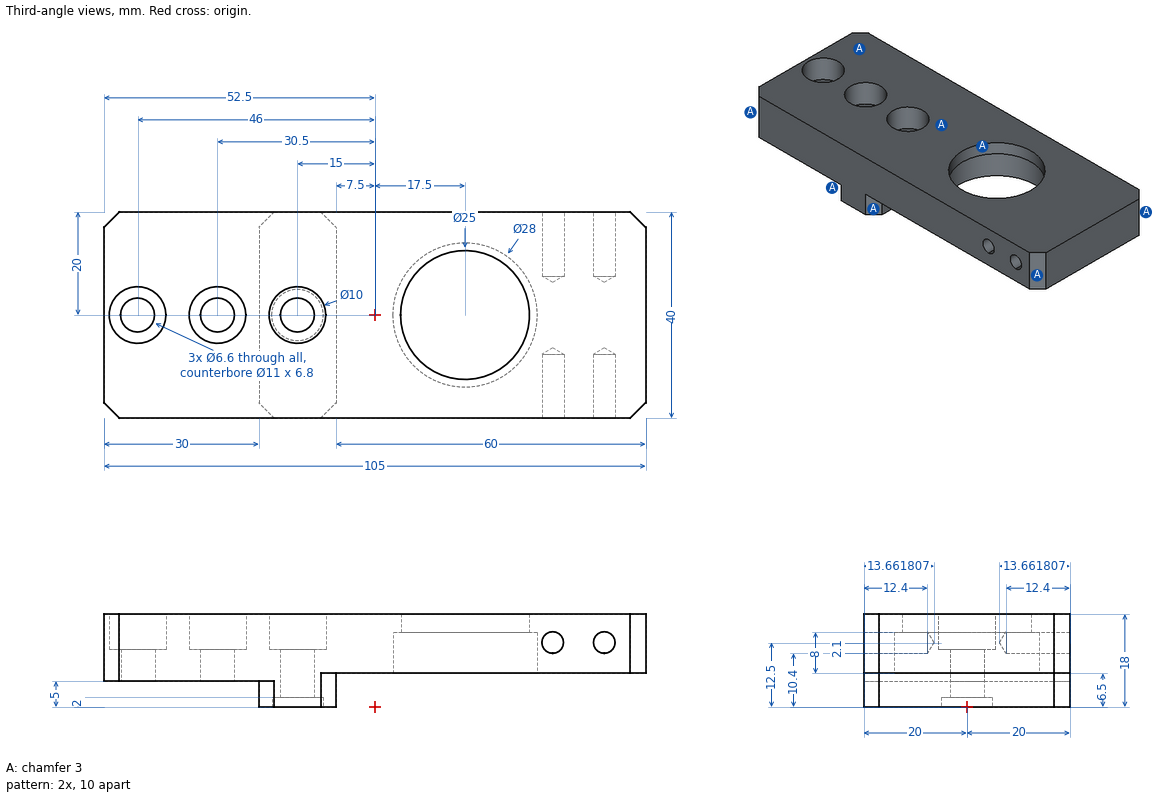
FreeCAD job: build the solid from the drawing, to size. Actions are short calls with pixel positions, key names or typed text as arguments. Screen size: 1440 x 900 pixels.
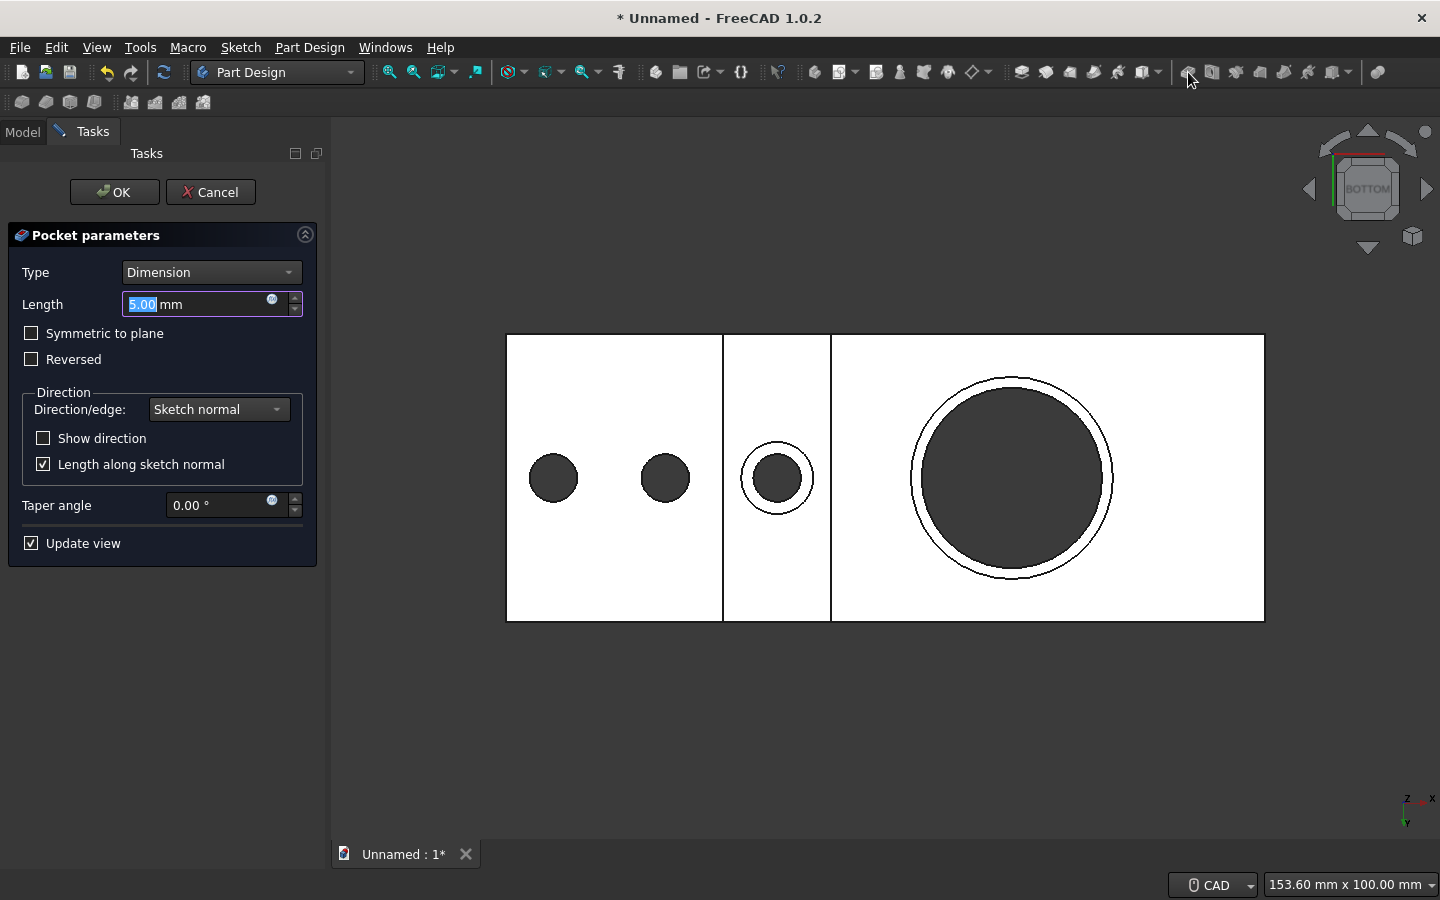
click(212, 272)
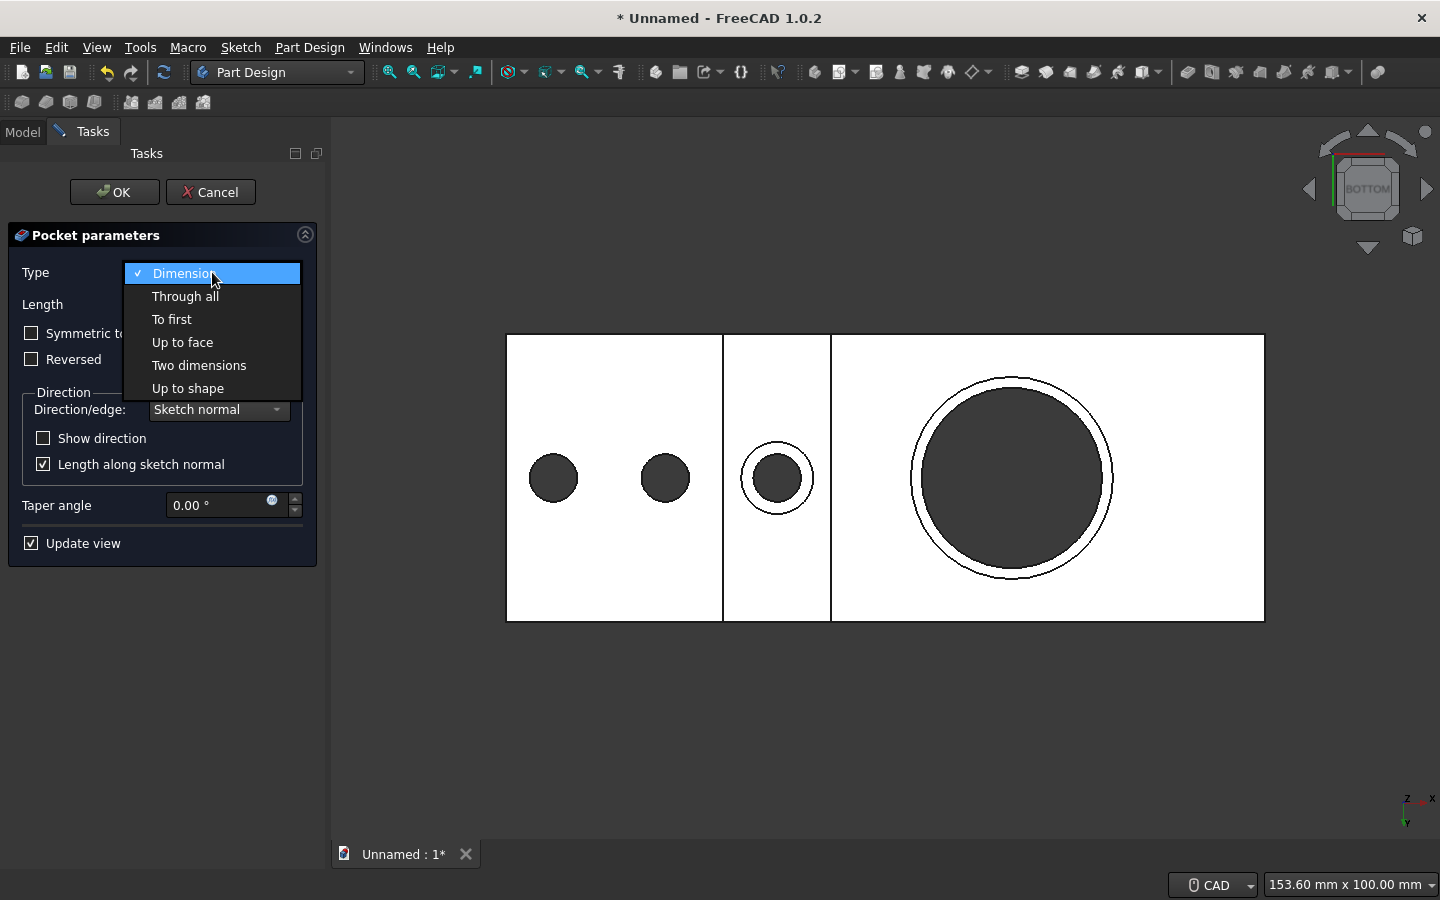
click(212, 296)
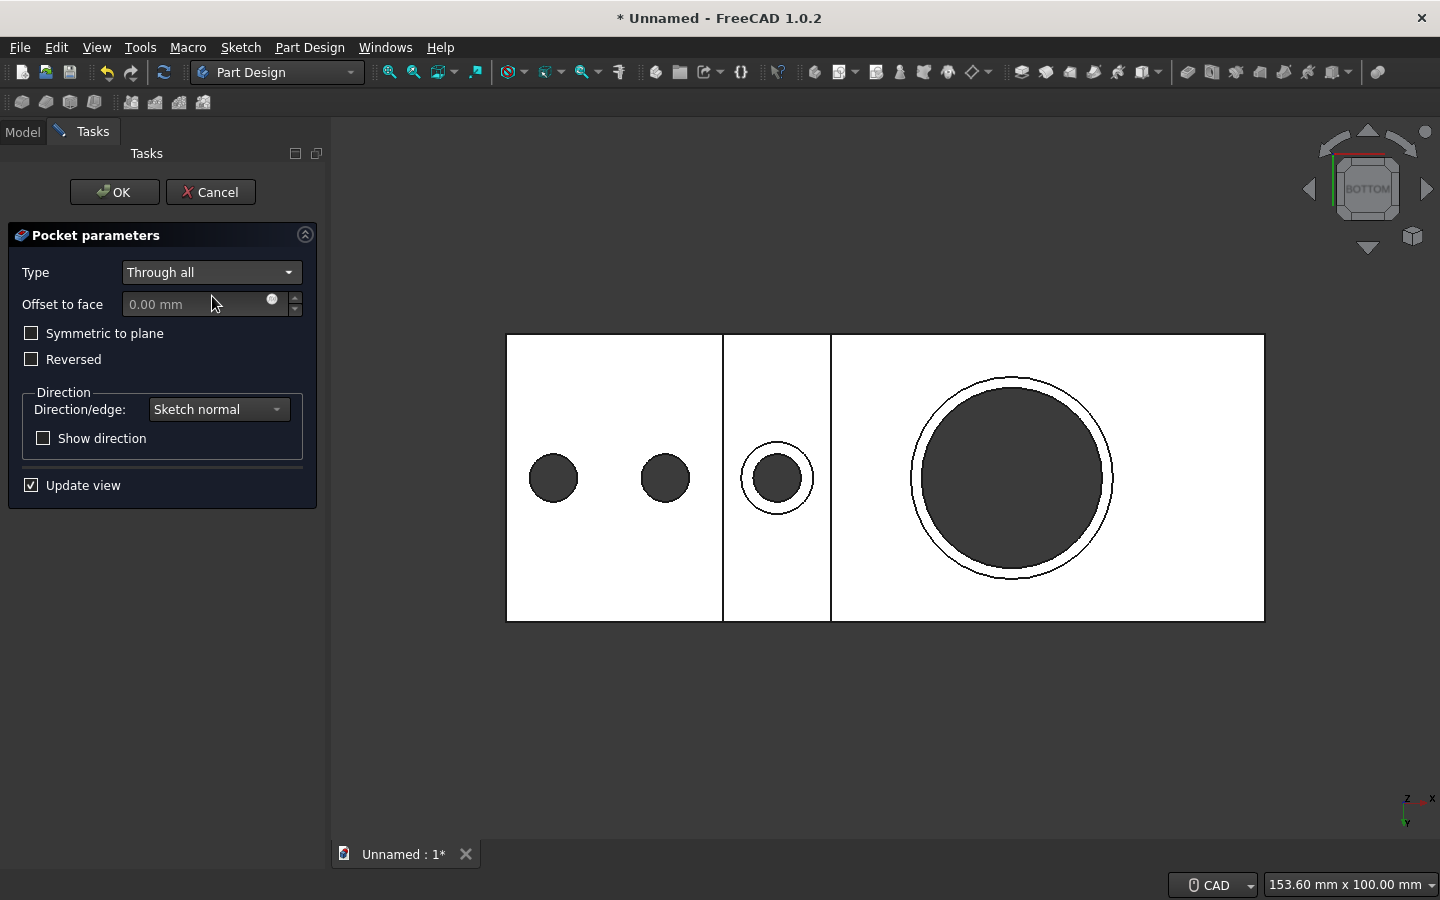
click(115, 192)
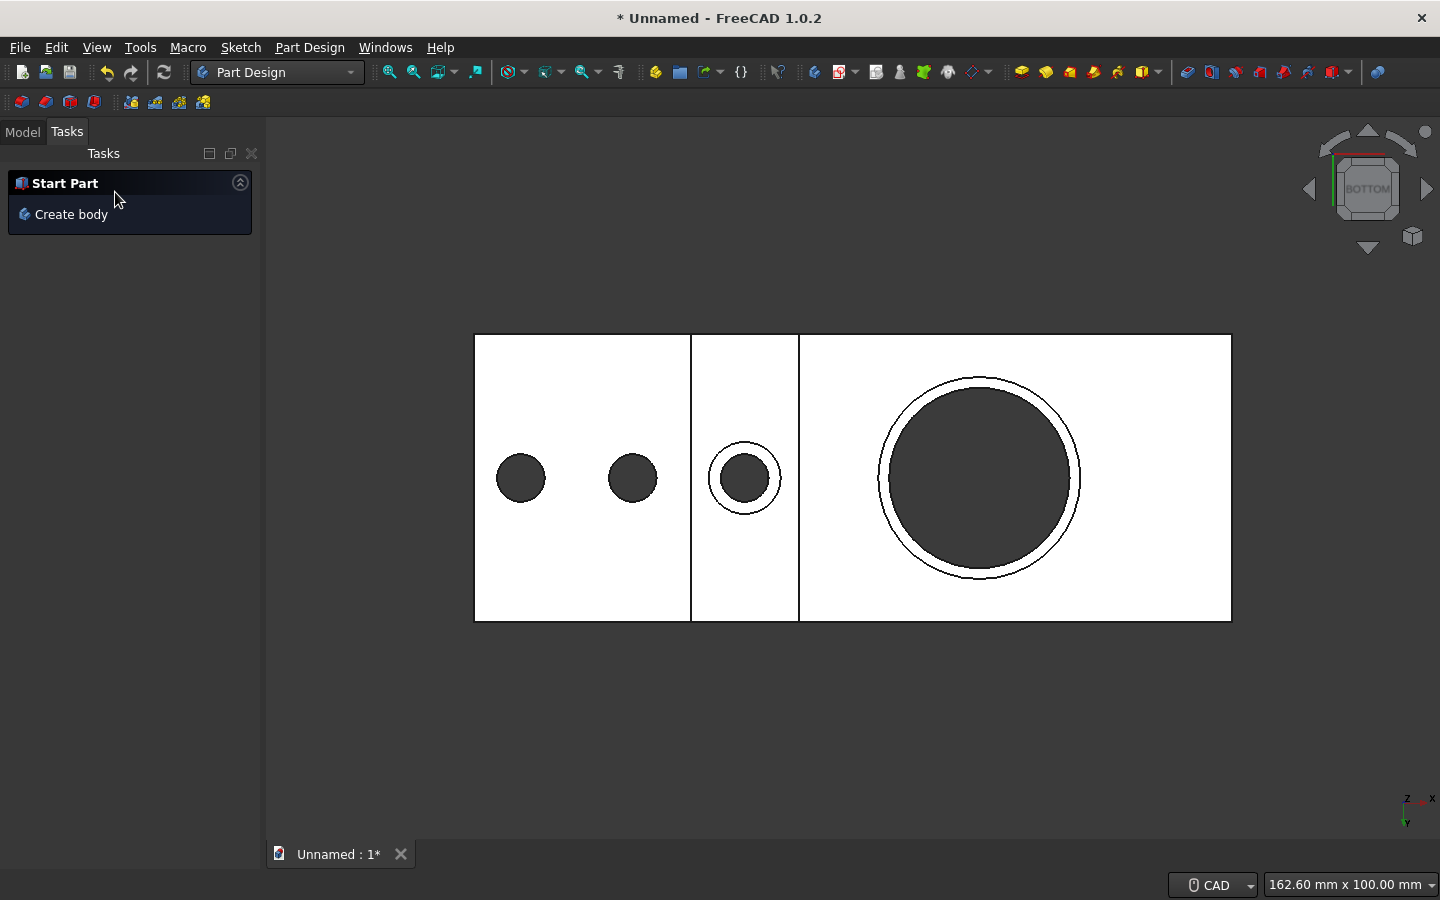
key(0)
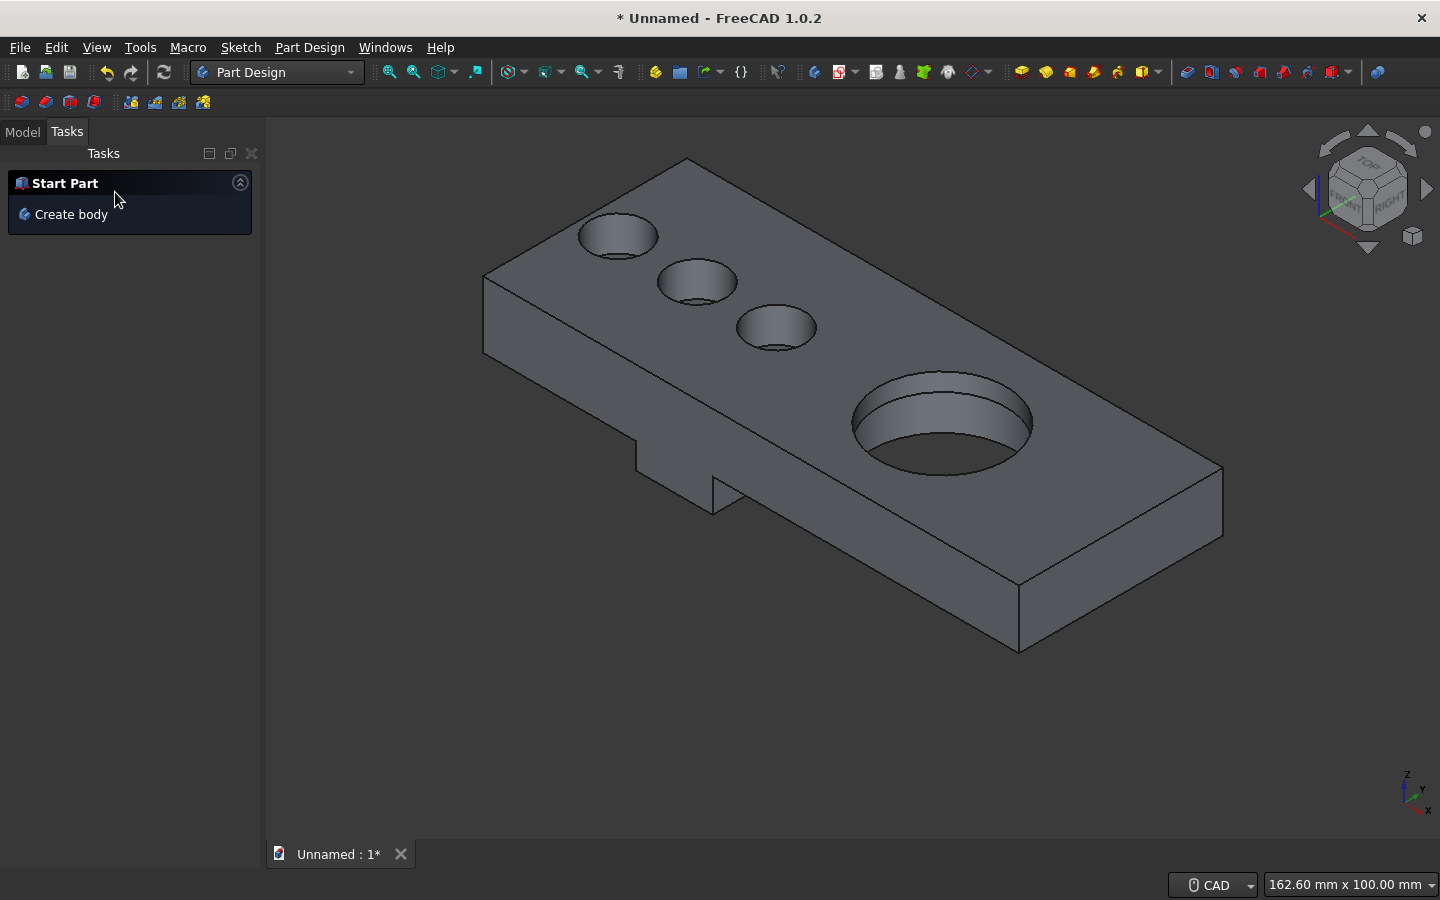
click(713, 495)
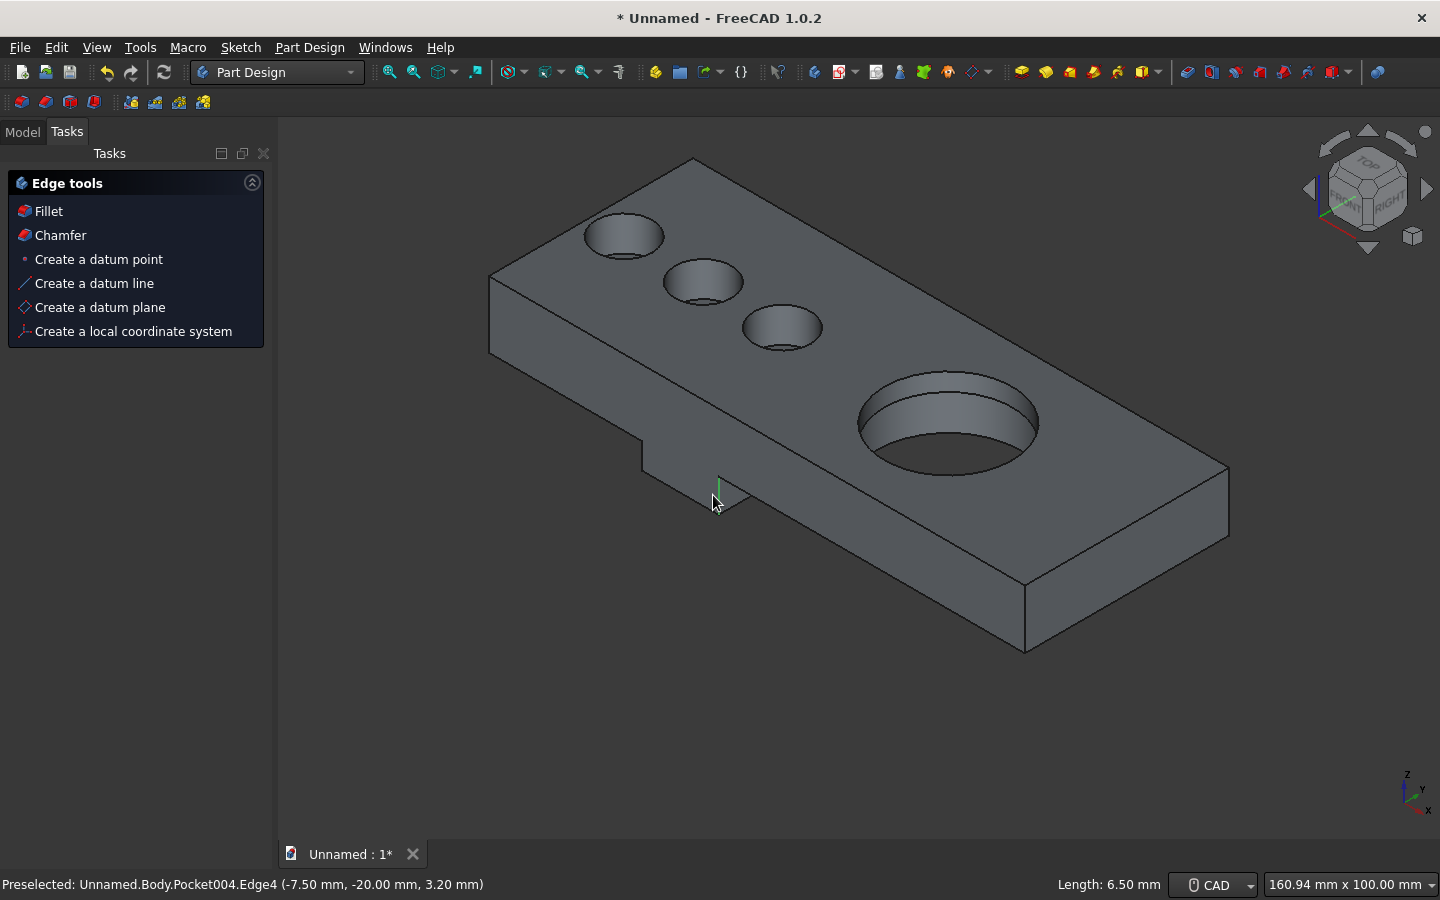
click(1025, 618, ctrl)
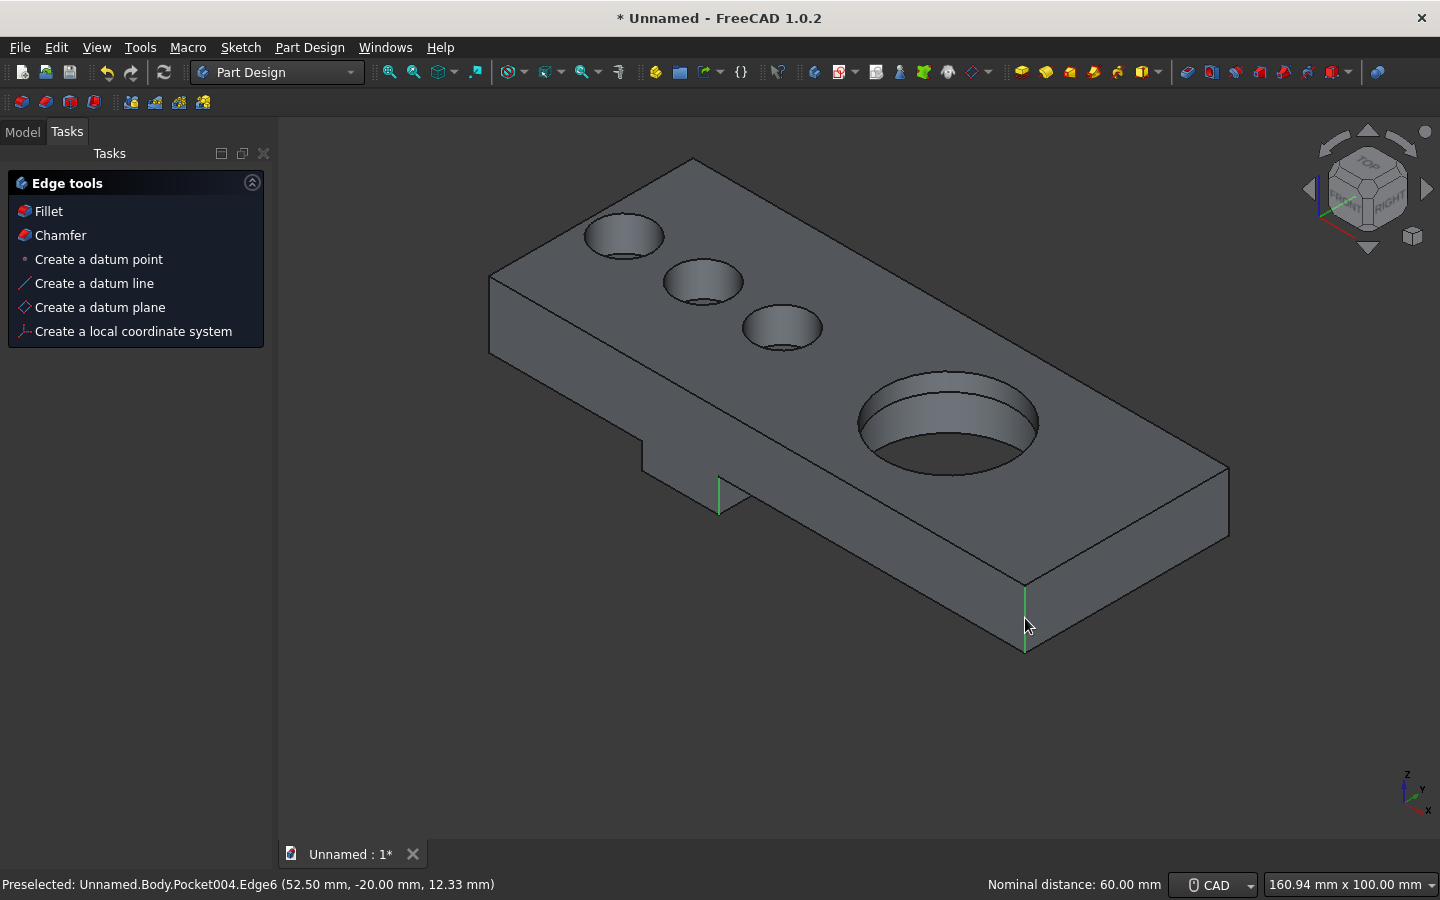
key(2)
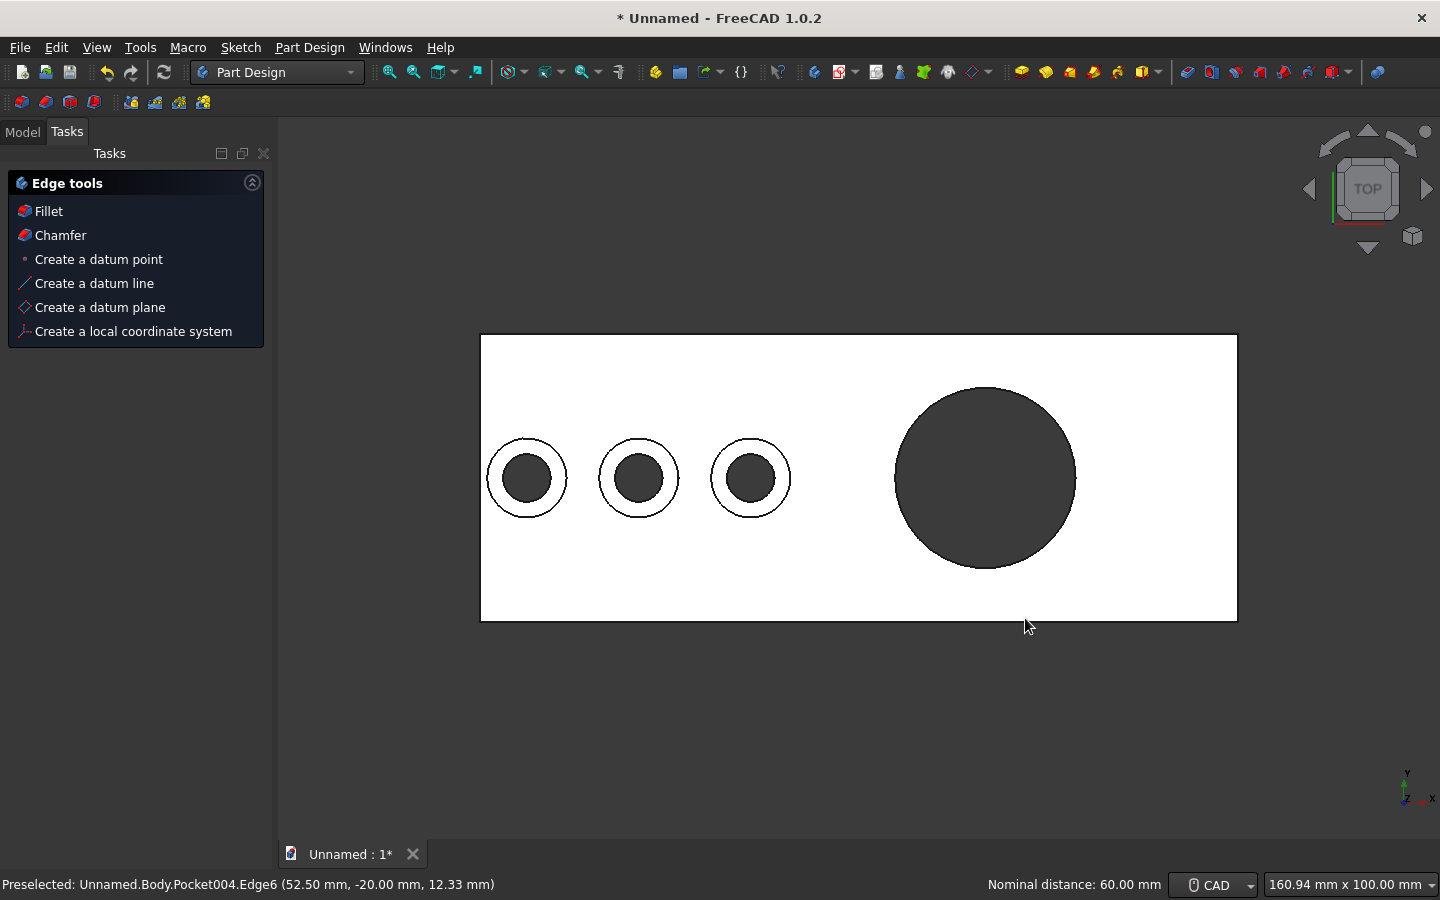
key(1)